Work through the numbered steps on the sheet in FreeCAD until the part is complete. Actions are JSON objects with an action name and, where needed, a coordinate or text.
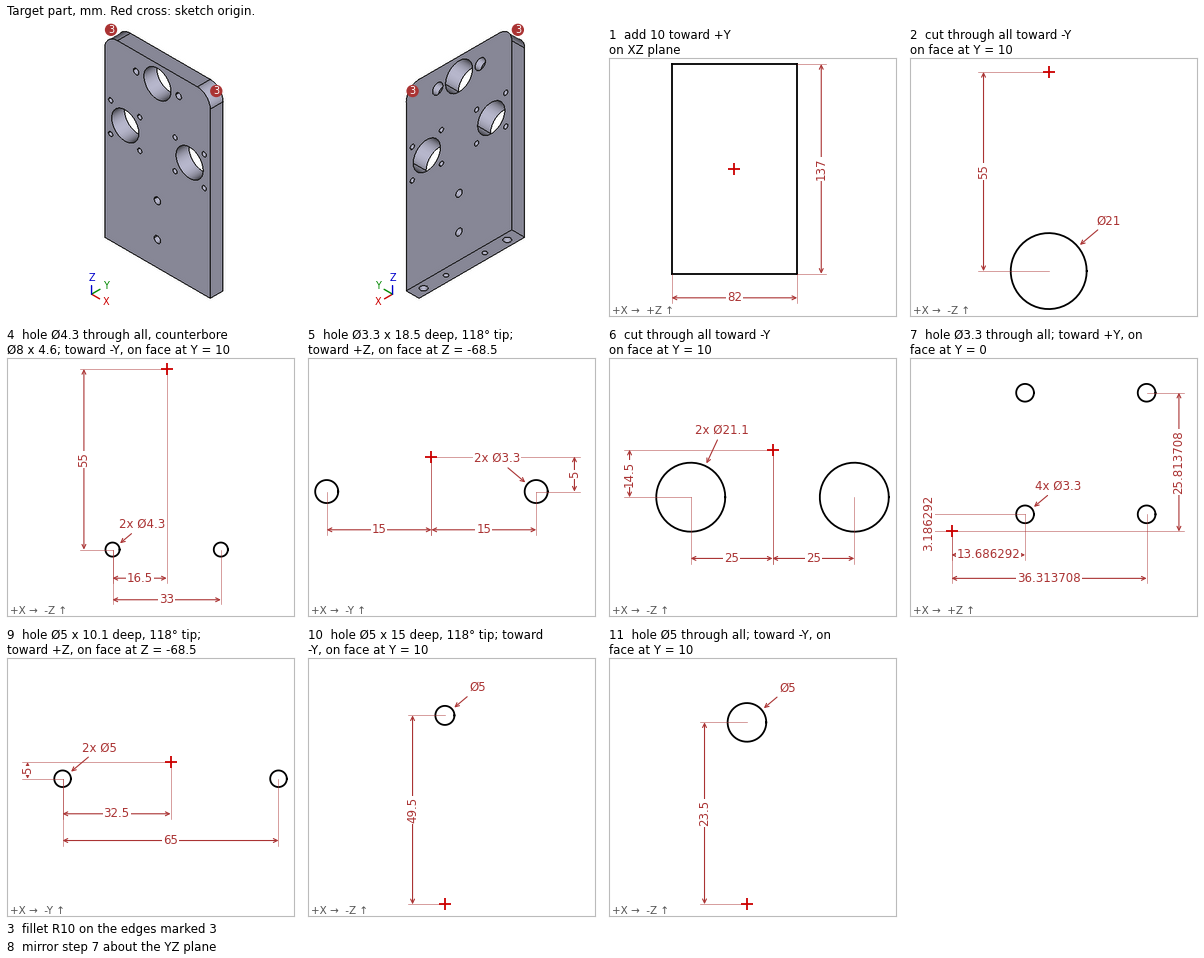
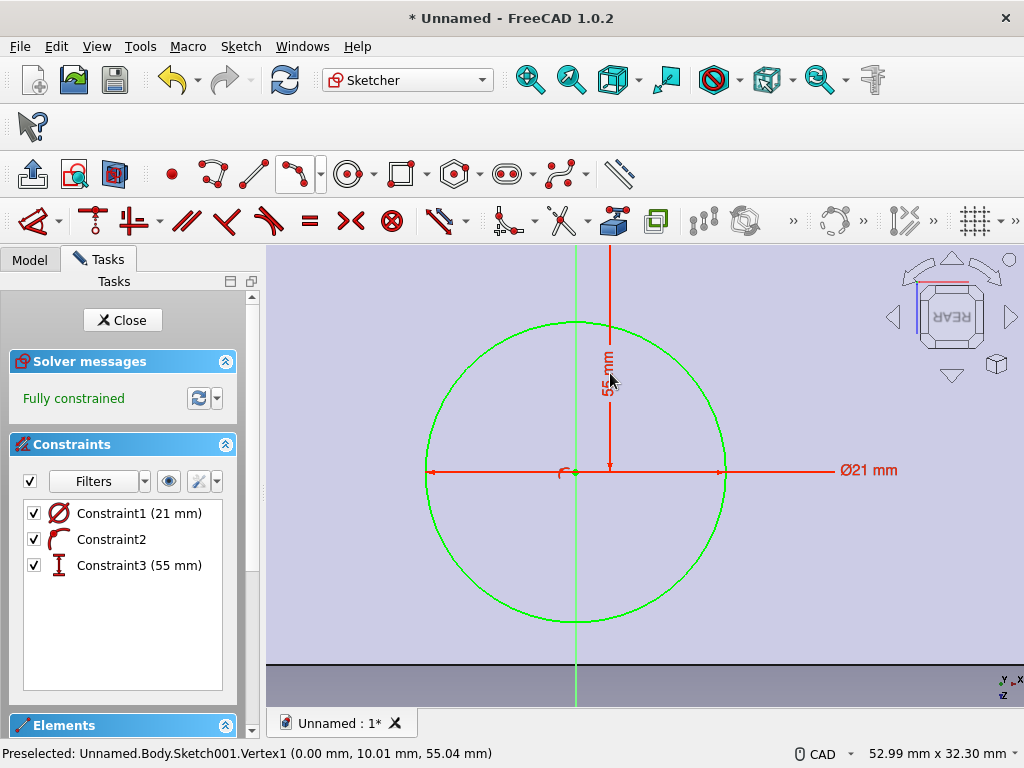
{"action": "left_click", "coordinate": [123, 320]}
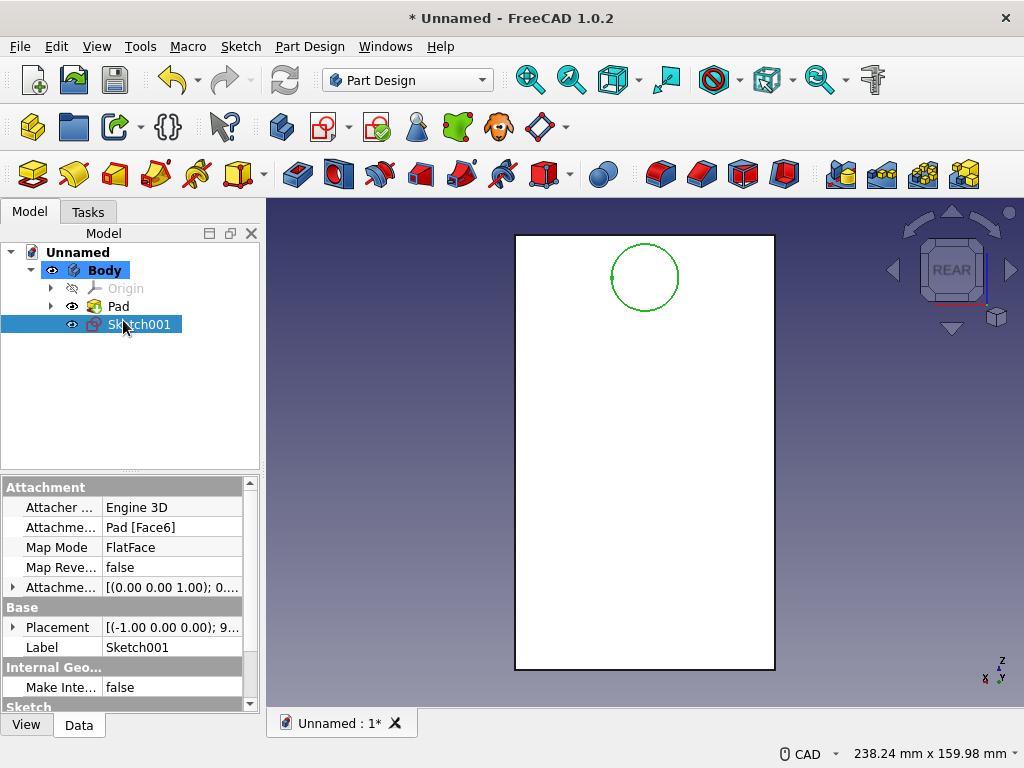
{"action": "left_click", "coordinate": [298, 174]}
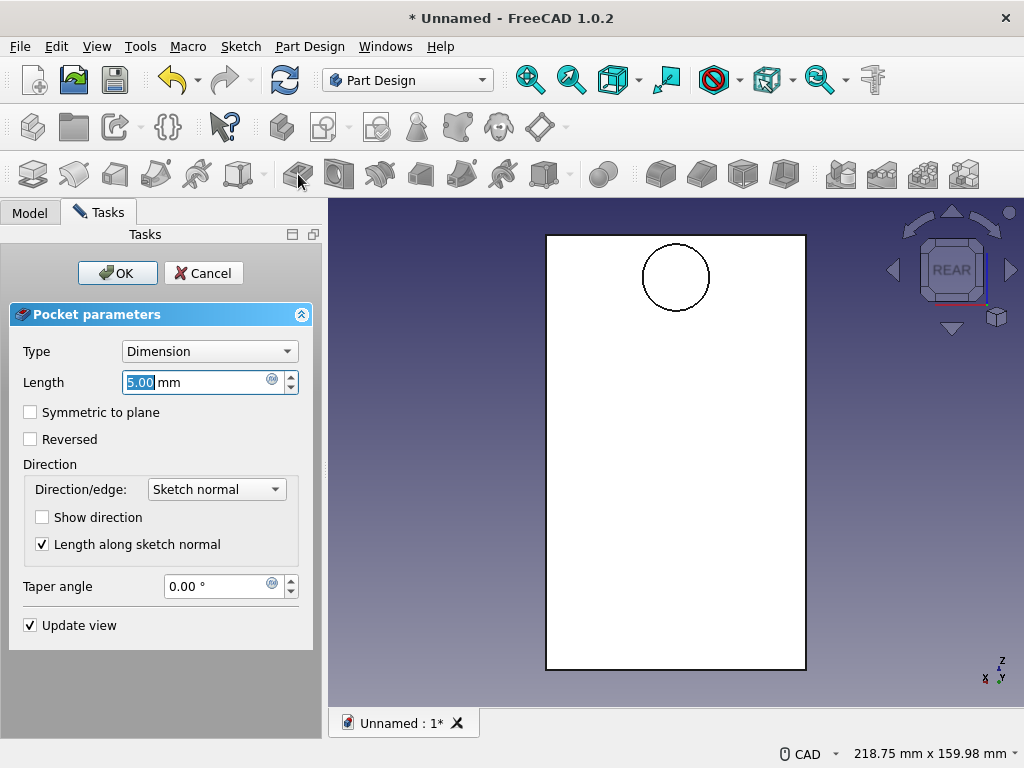
{"action": "left_click", "coordinate": [210, 352]}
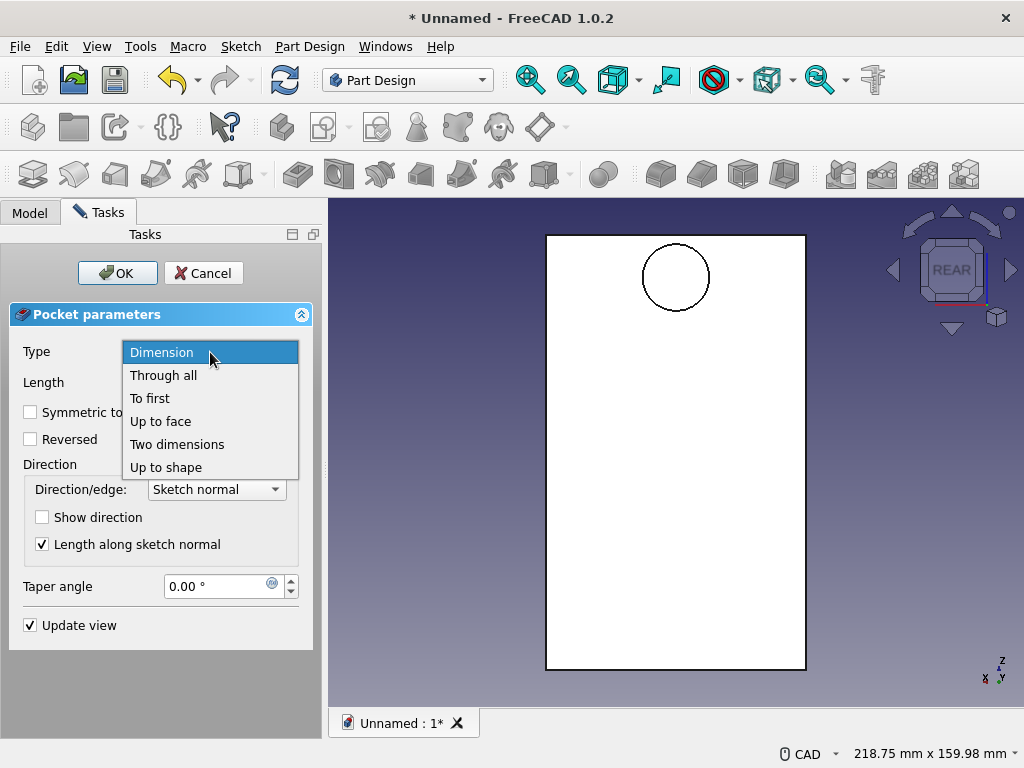
{"action": "left_click", "coordinate": [208, 376]}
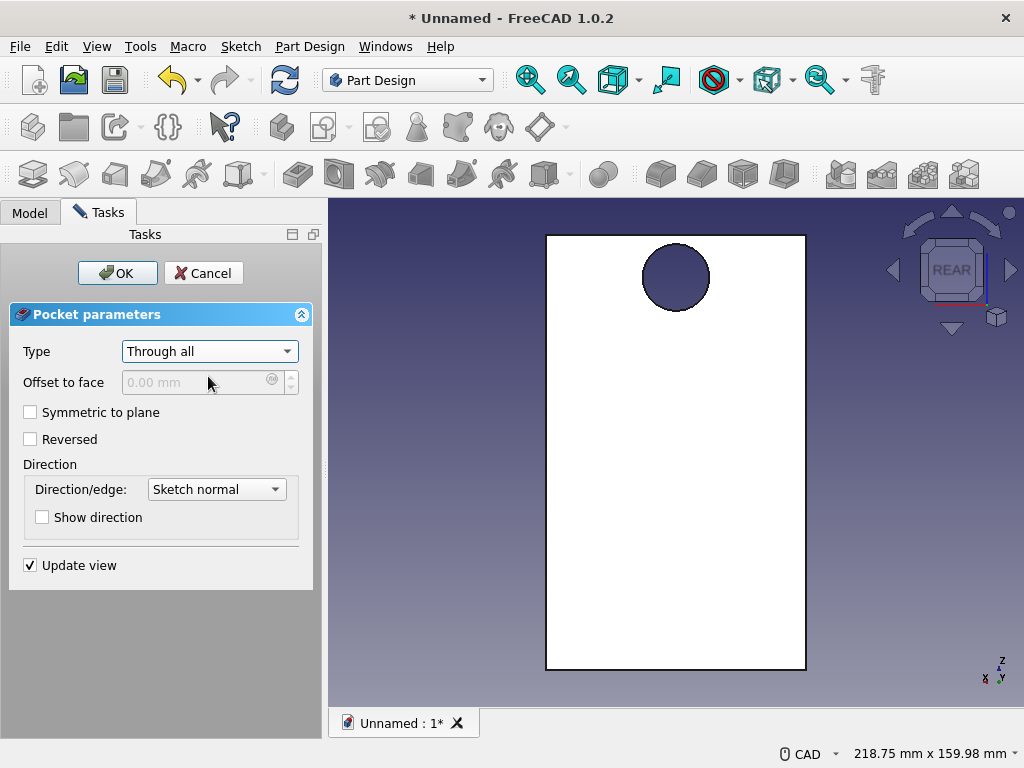
{"action": "left_click", "coordinate": [118, 273]}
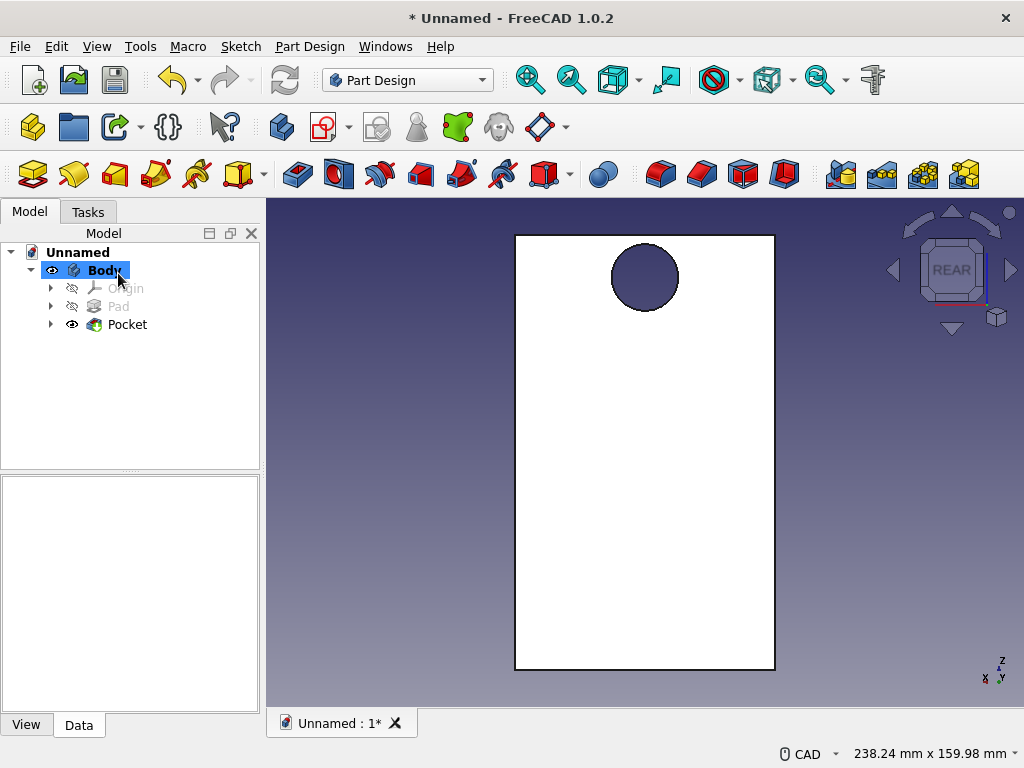
{"action": "key", "text": "0"}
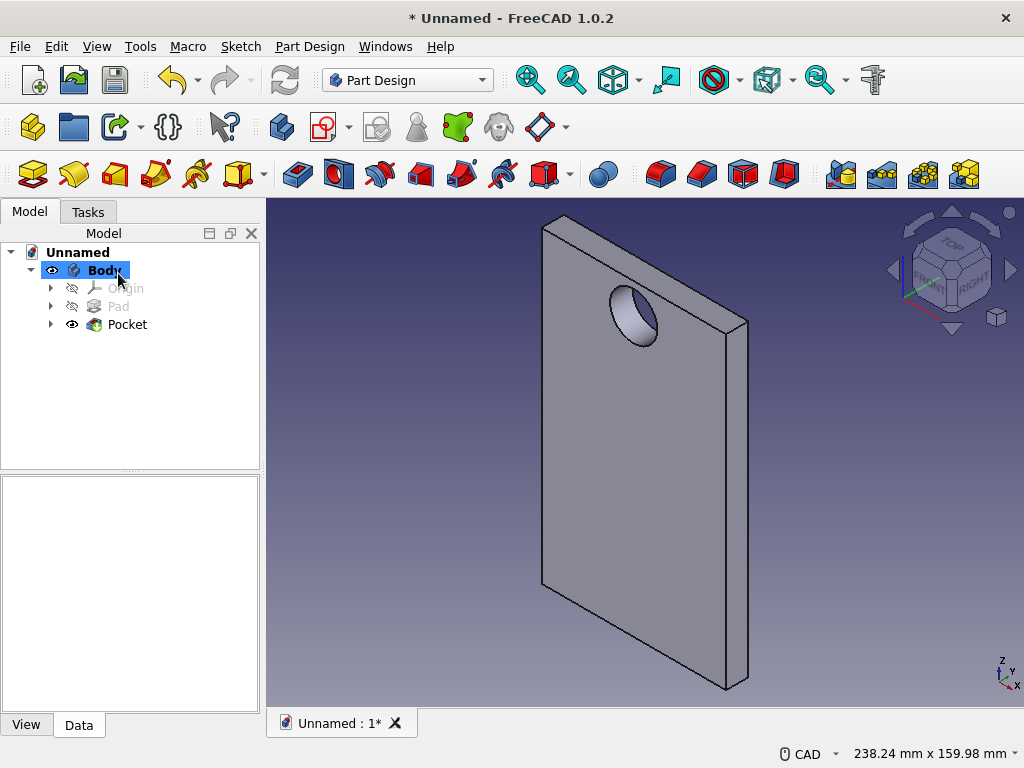
{"action": "left_click", "coordinate": [737, 327]}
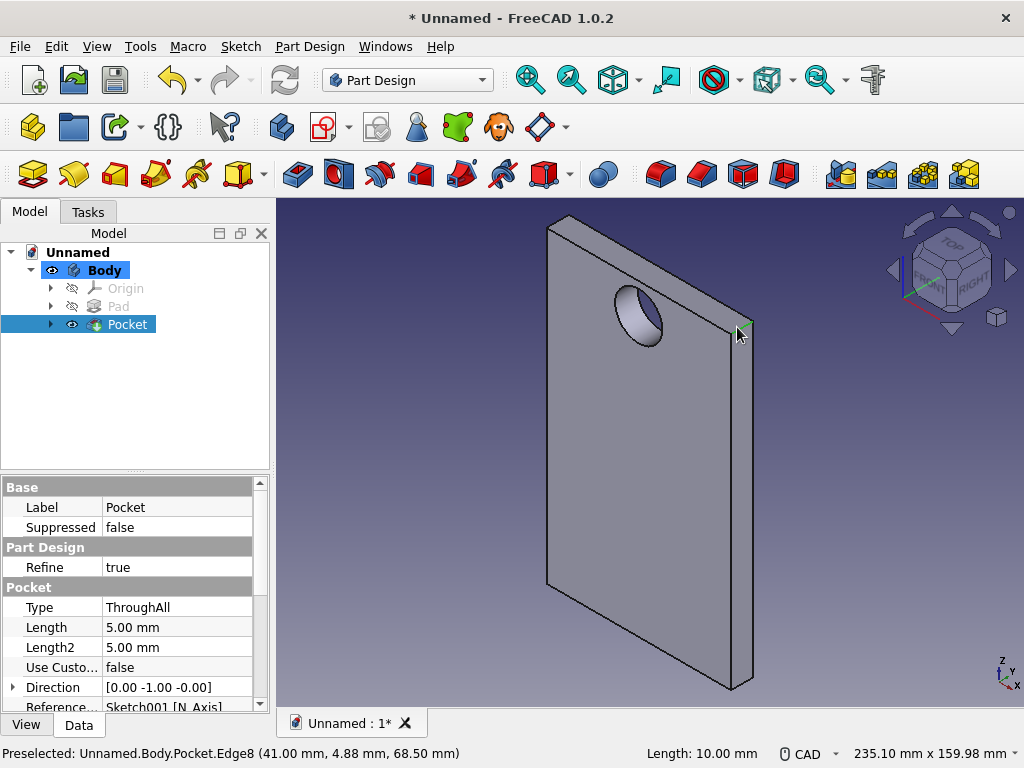
{"action": "key", "text": "2"}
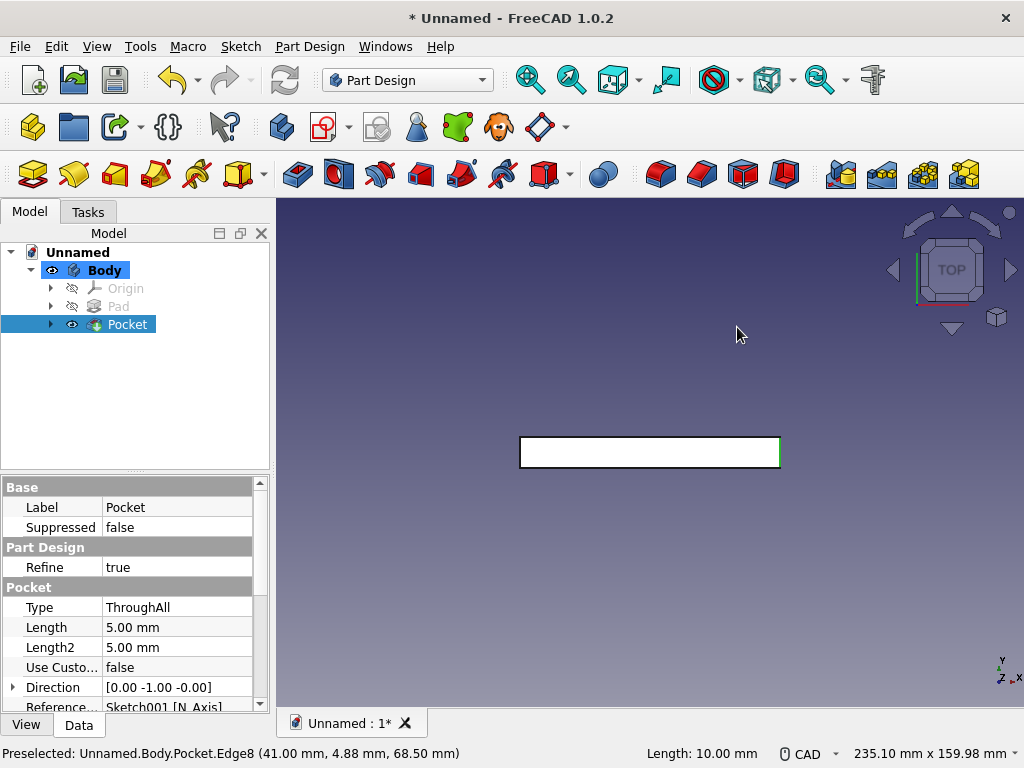
{"action": "key", "text": "v f"}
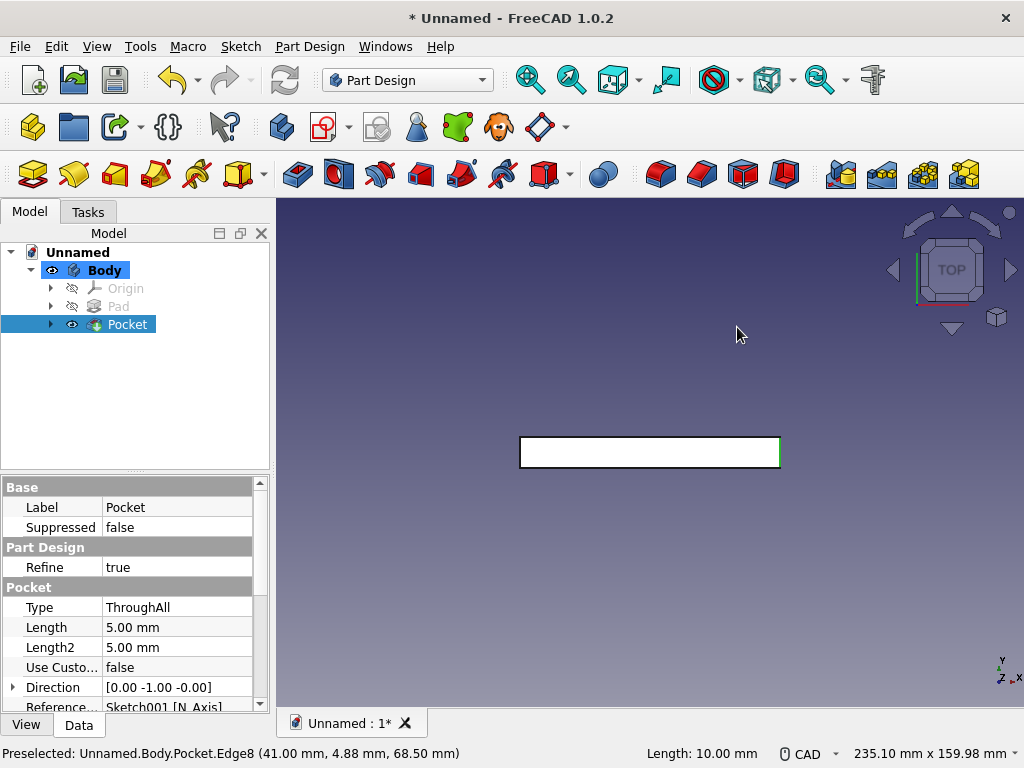
{"action": "left_click", "coordinate": [520, 451], "text": "ctrl"}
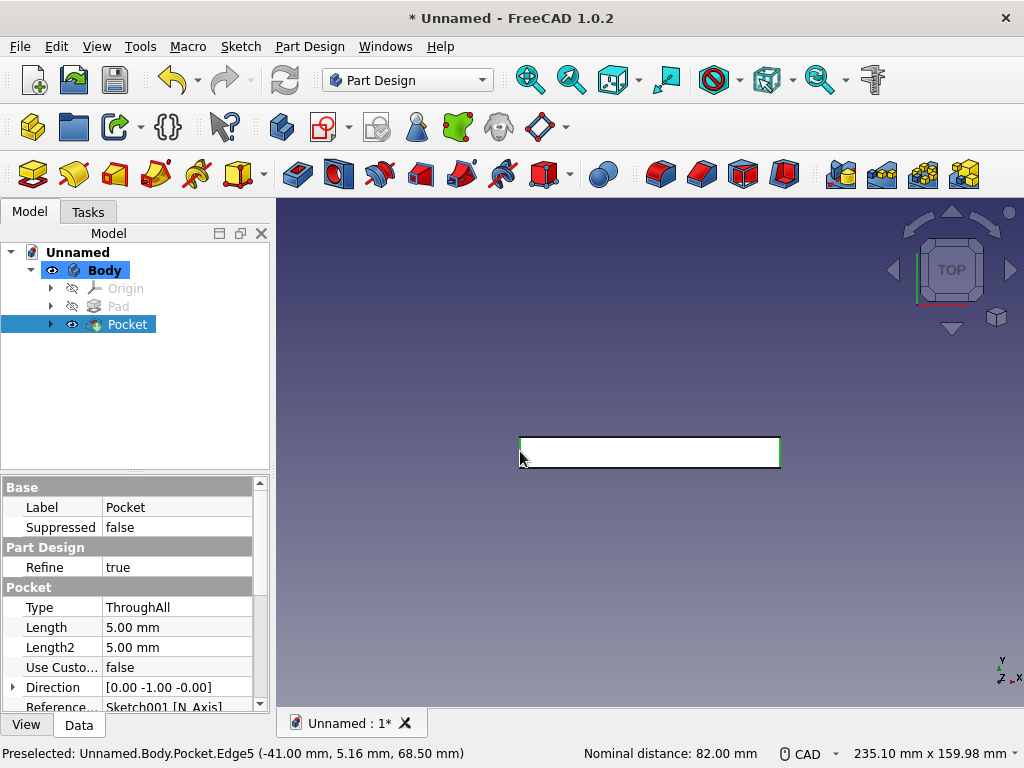
{"action": "left_click", "coordinate": [661, 174]}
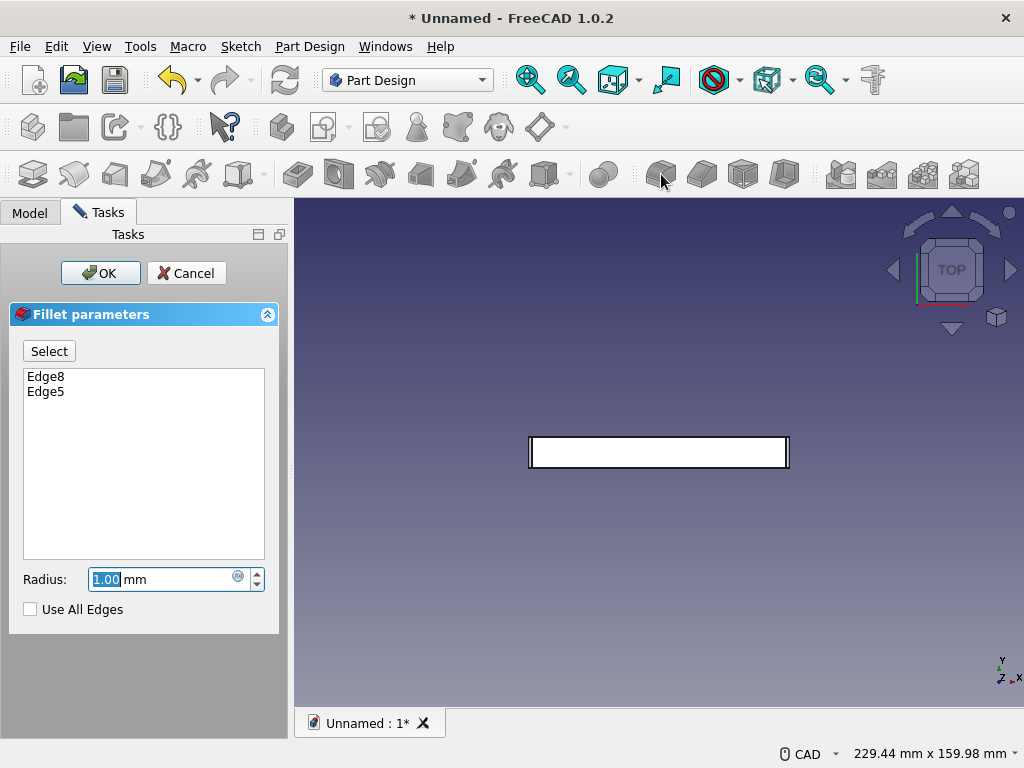
{"action": "type", "text": "10"}
{"action": "key", "text": "Tab"}